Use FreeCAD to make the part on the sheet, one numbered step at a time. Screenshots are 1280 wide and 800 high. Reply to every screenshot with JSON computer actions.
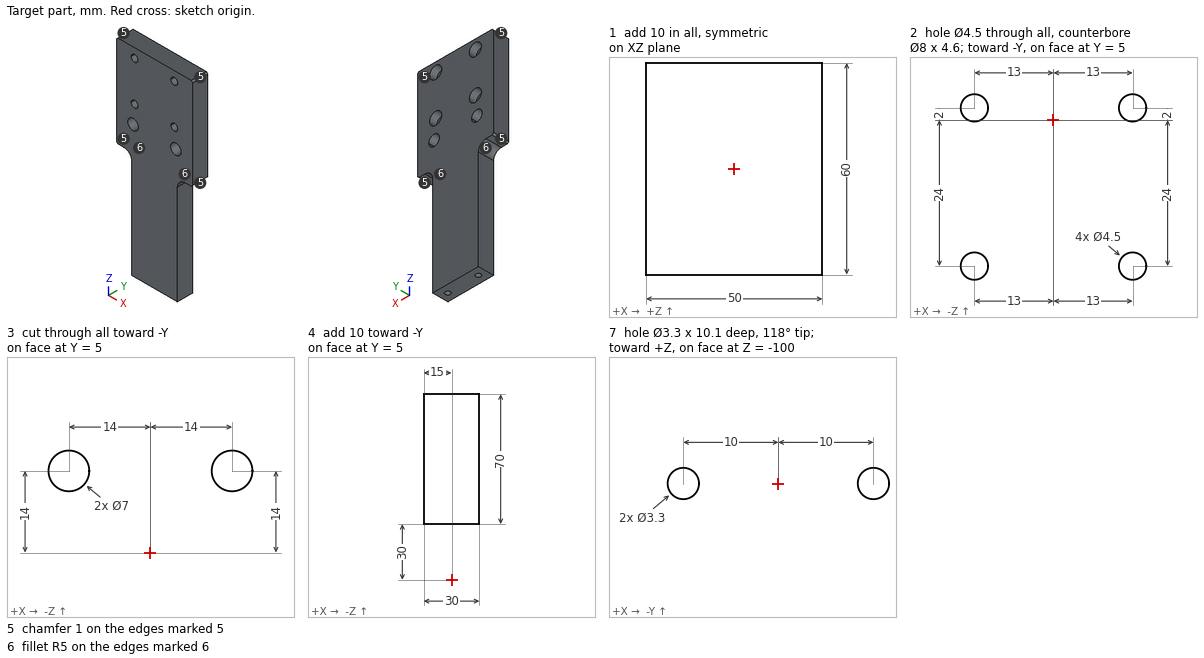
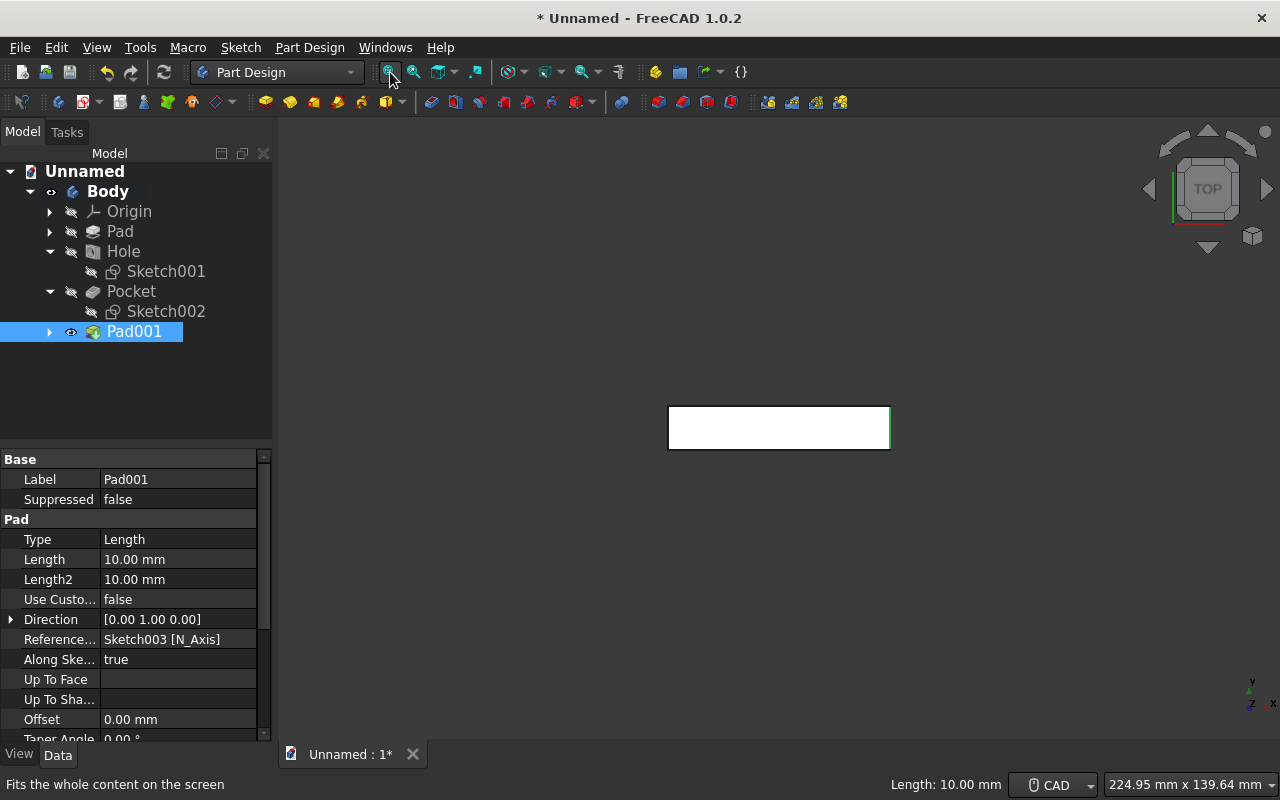
{"action": "left_click", "coordinate": [668, 427], "text": "ctrl"}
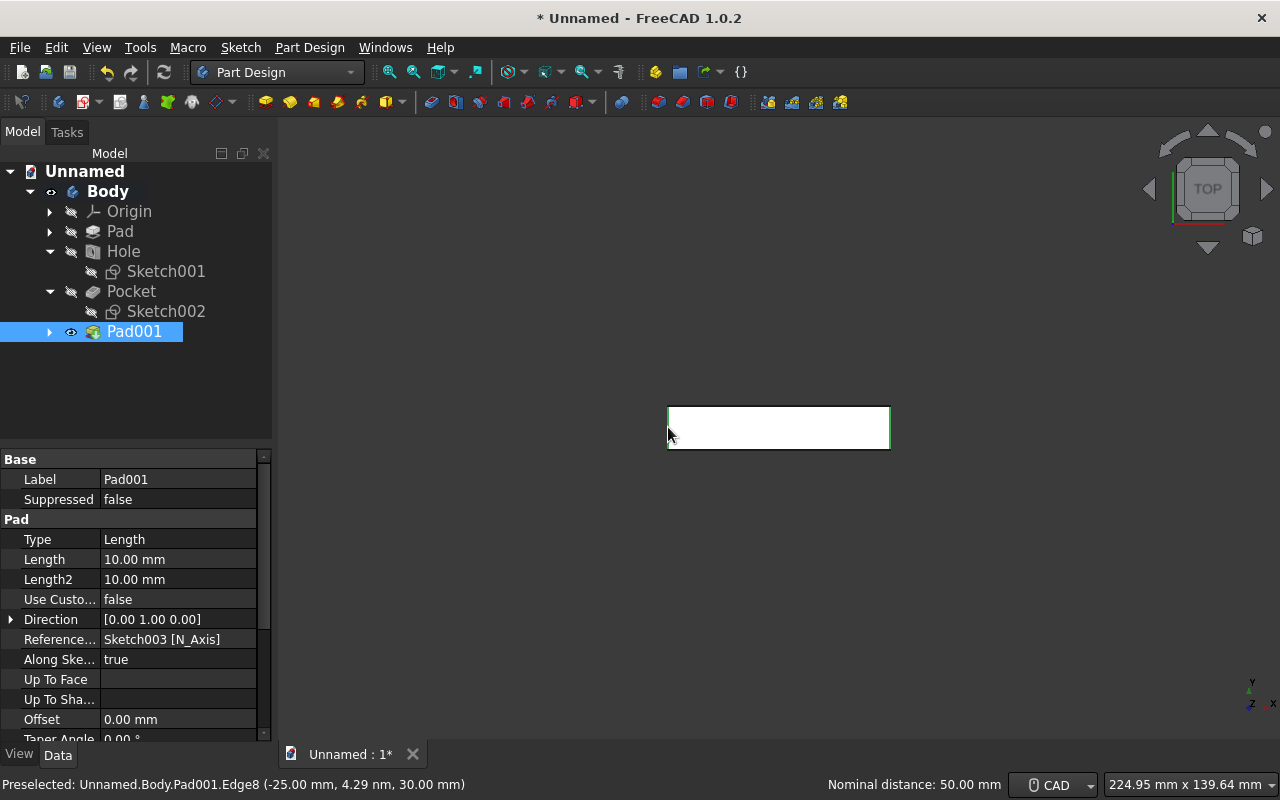
{"action": "key", "text": "1"}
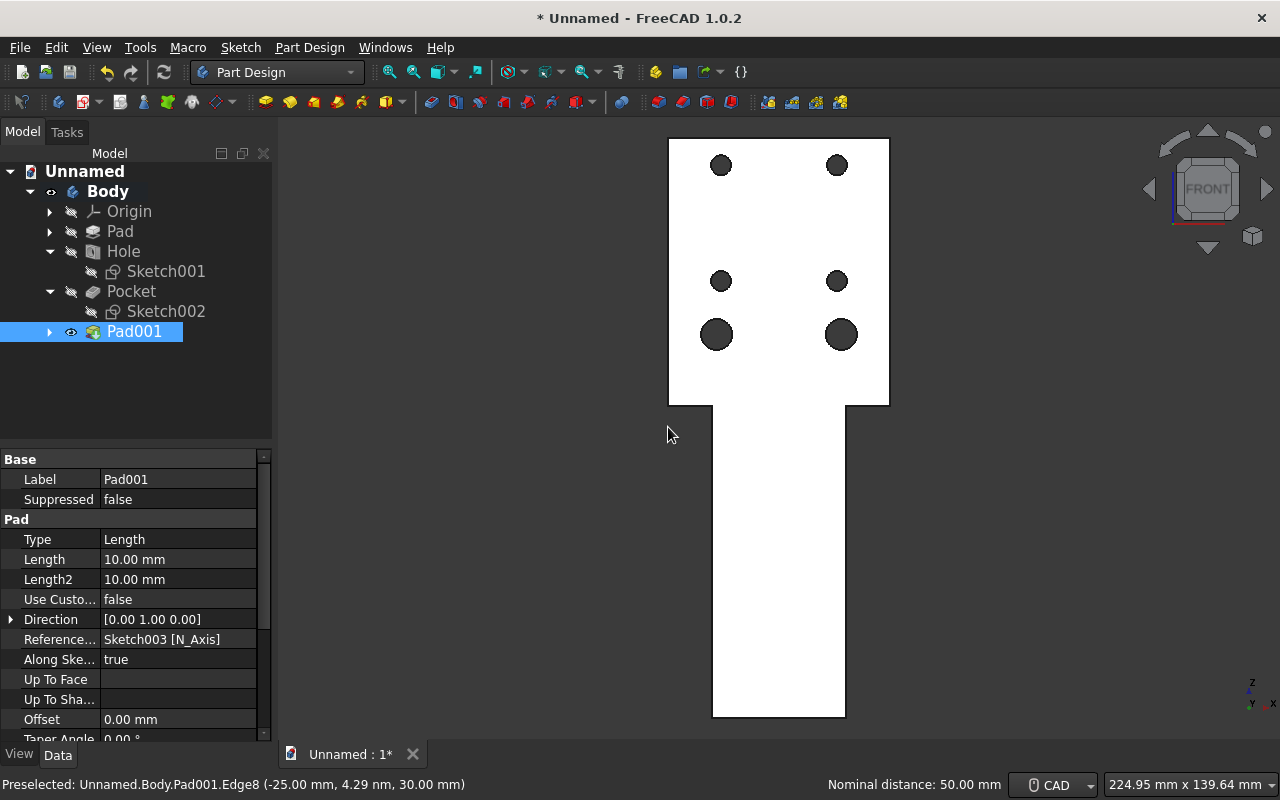
{"action": "key", "text": "3"}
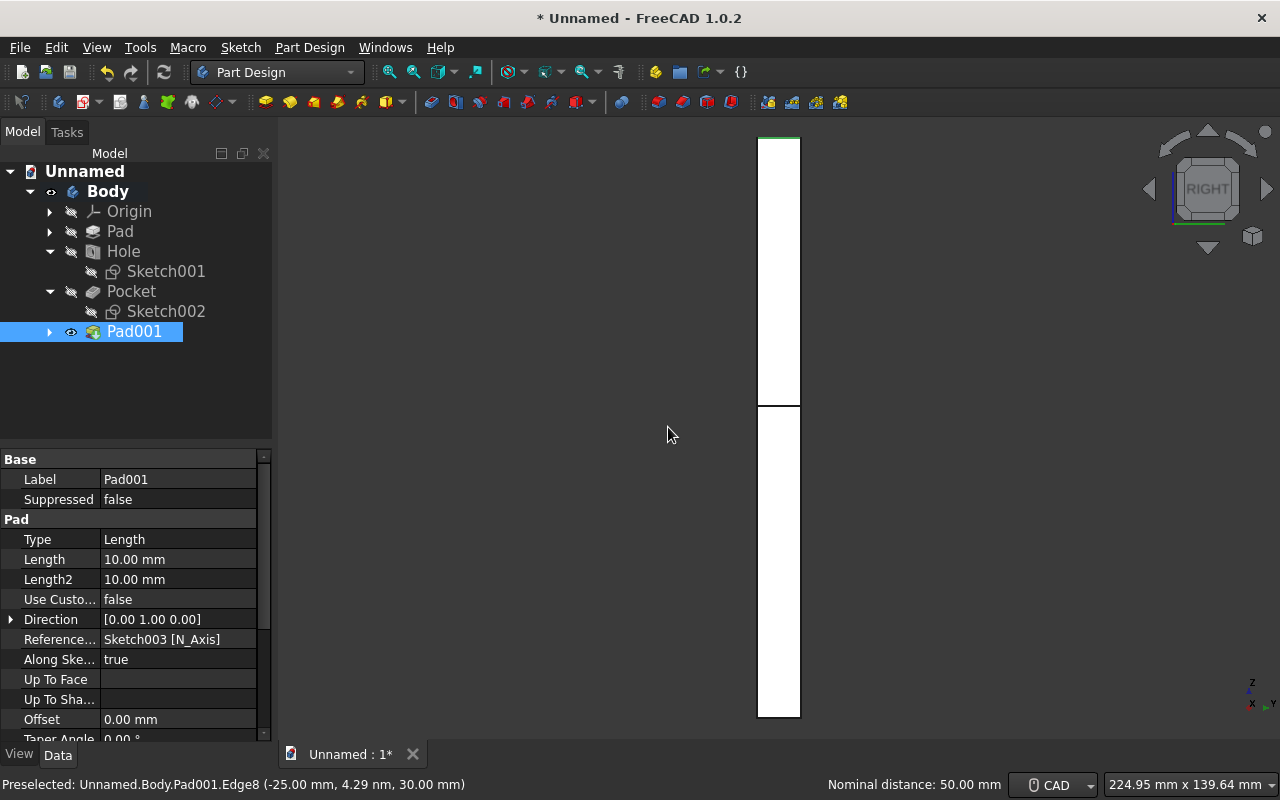
{"action": "left_click", "coordinate": [779, 405], "text": "ctrl"}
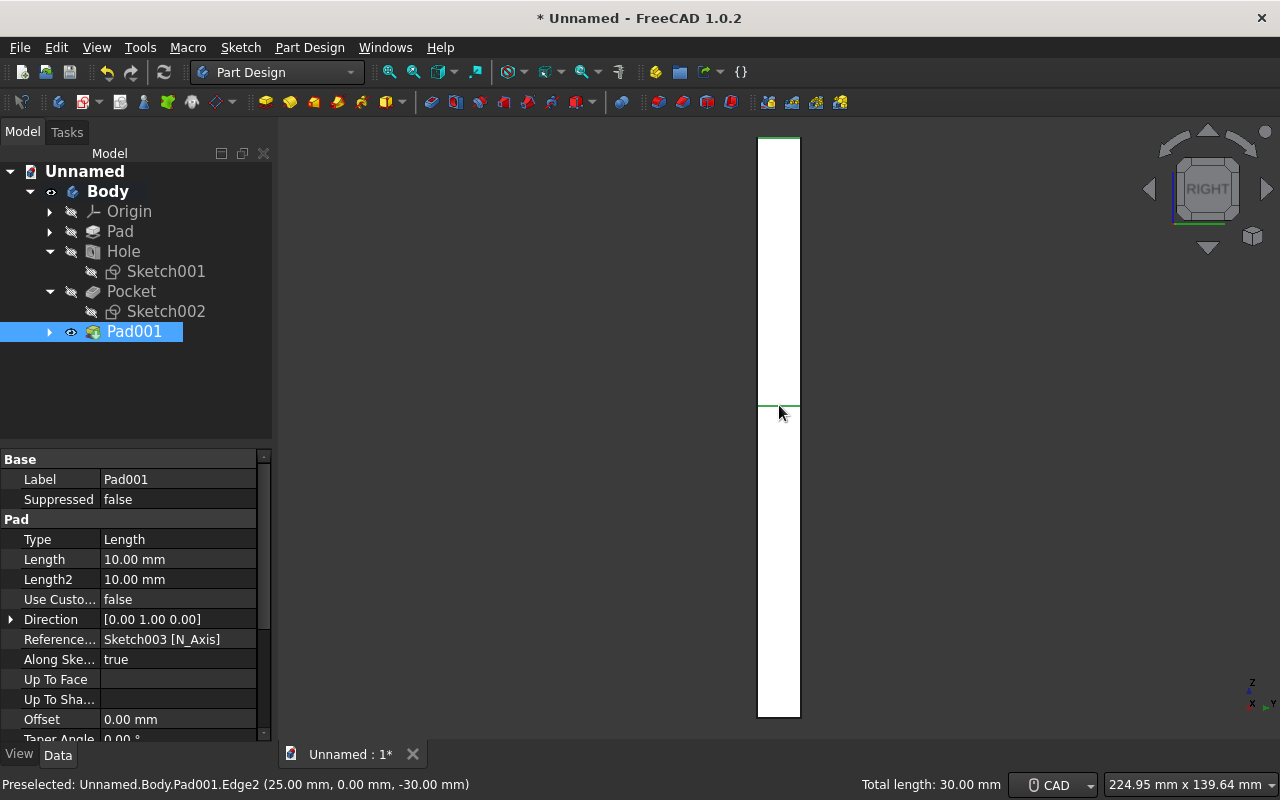
{"action": "key", "text": "5"}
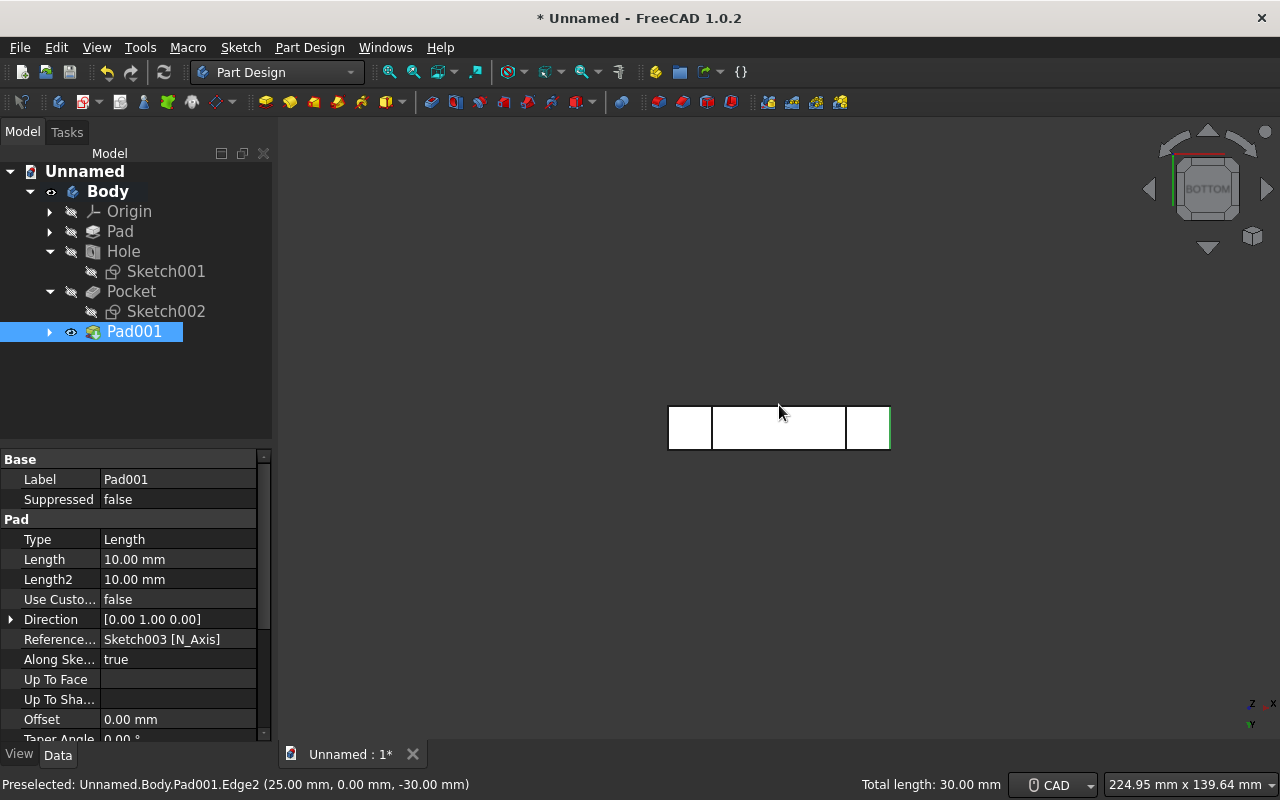
{"action": "left_click", "coordinate": [390, 72]}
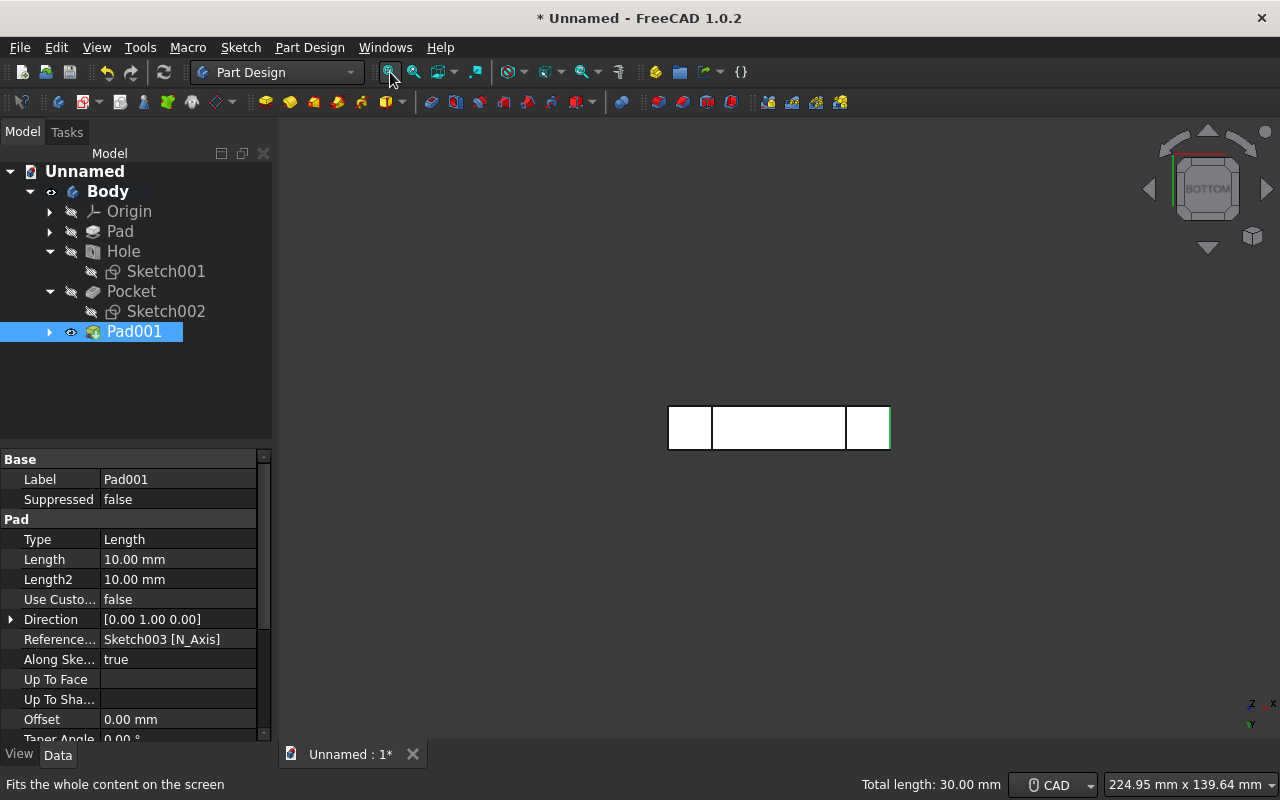
{"action": "left_click", "coordinate": [668, 427], "text": "ctrl"}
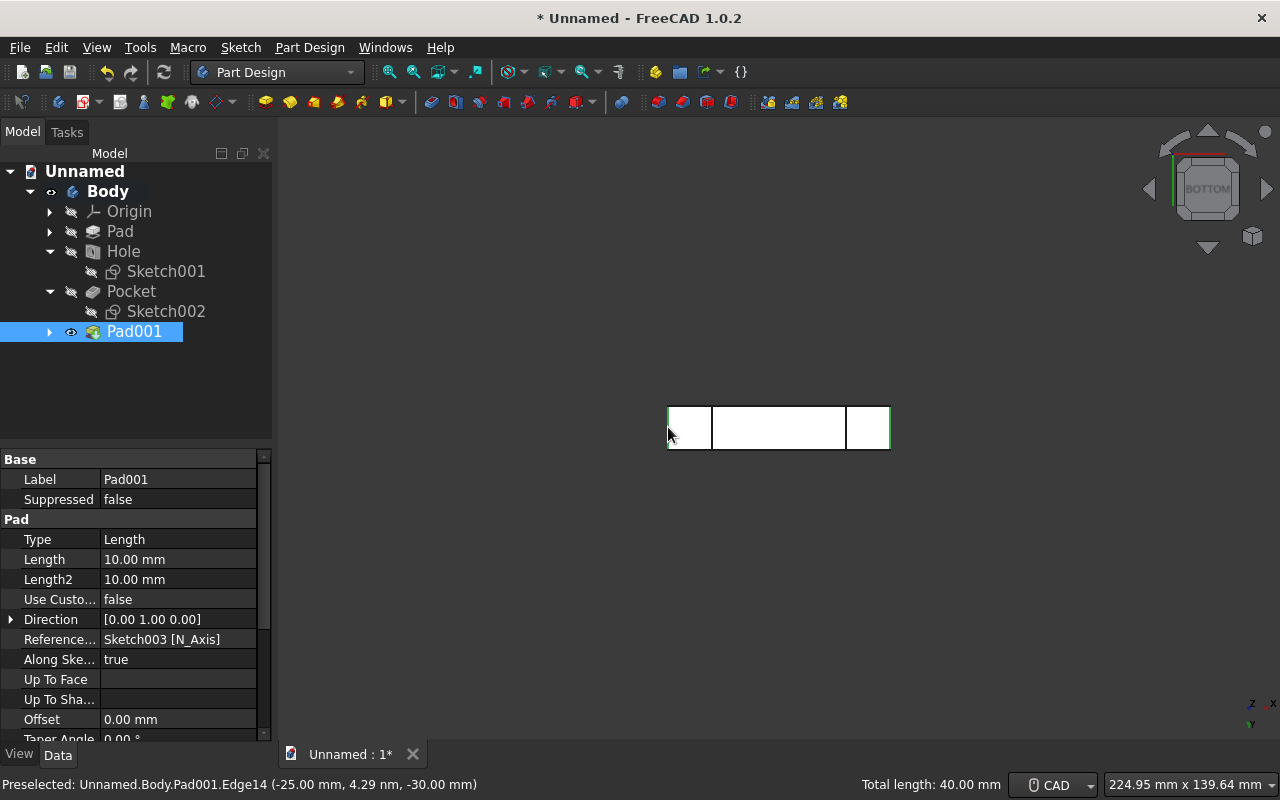
{"action": "left_click", "coordinate": [684, 102]}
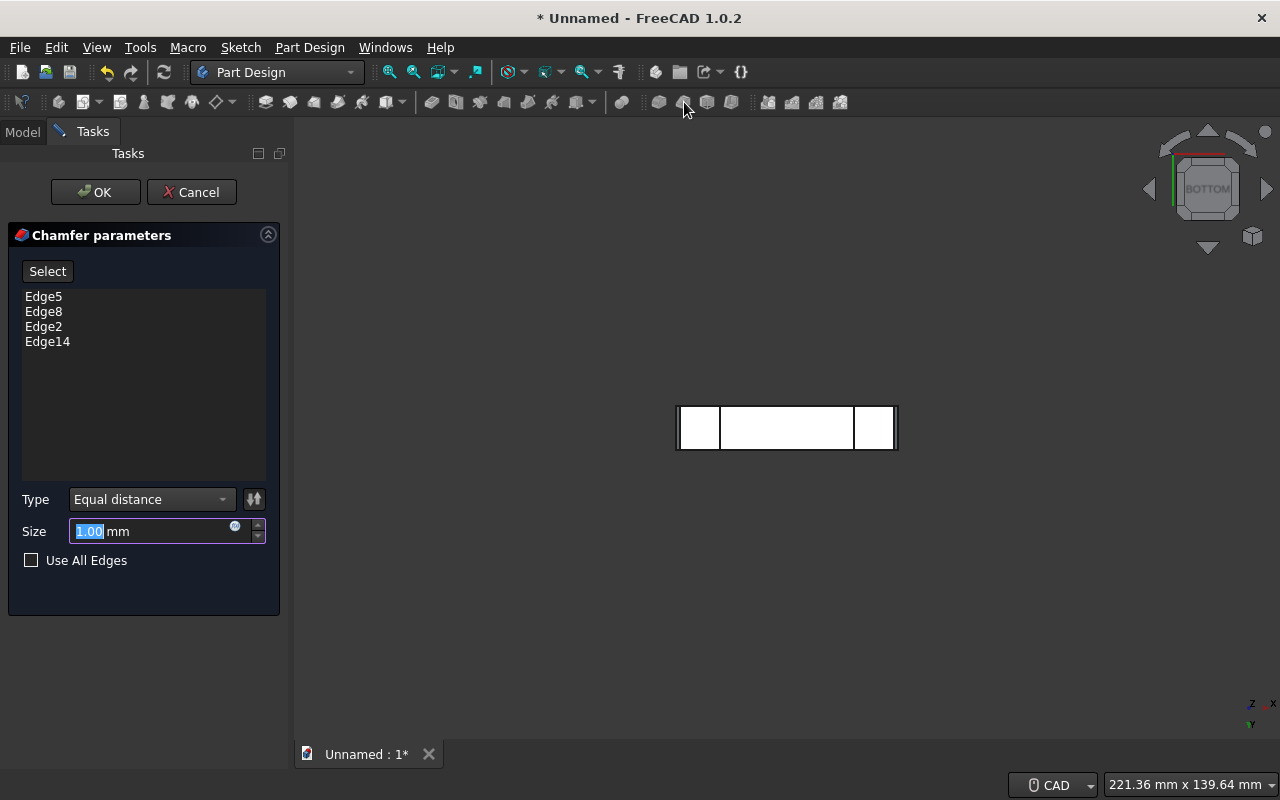
{"action": "type", "text": "1"}
{"action": "key", "text": "Tab"}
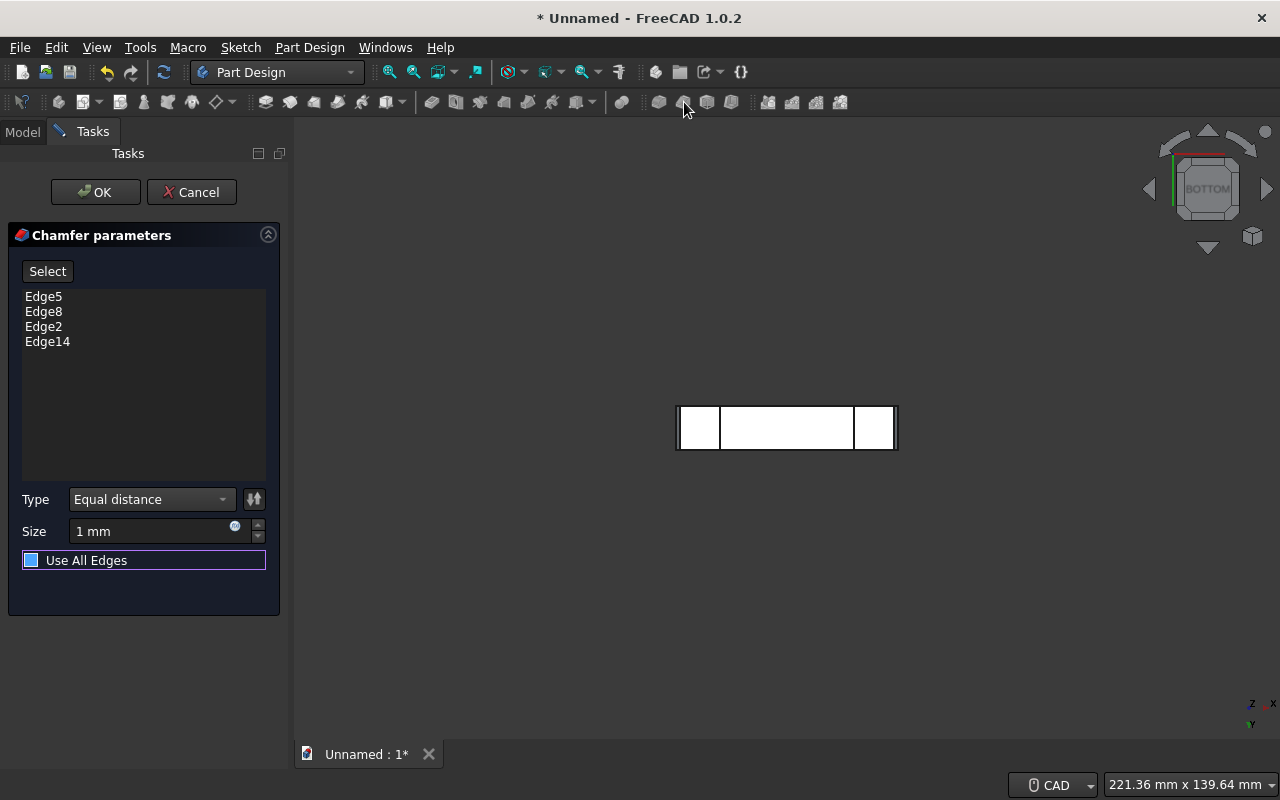
{"action": "left_click", "coordinate": [96, 192]}